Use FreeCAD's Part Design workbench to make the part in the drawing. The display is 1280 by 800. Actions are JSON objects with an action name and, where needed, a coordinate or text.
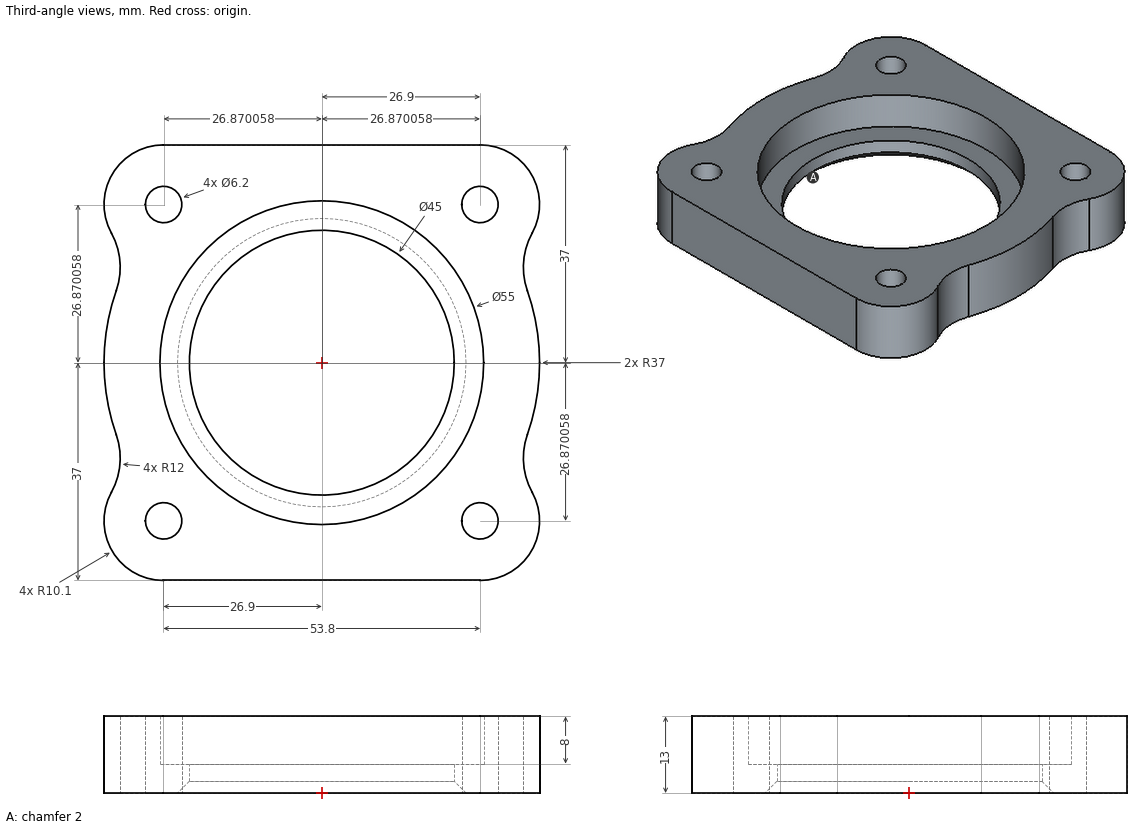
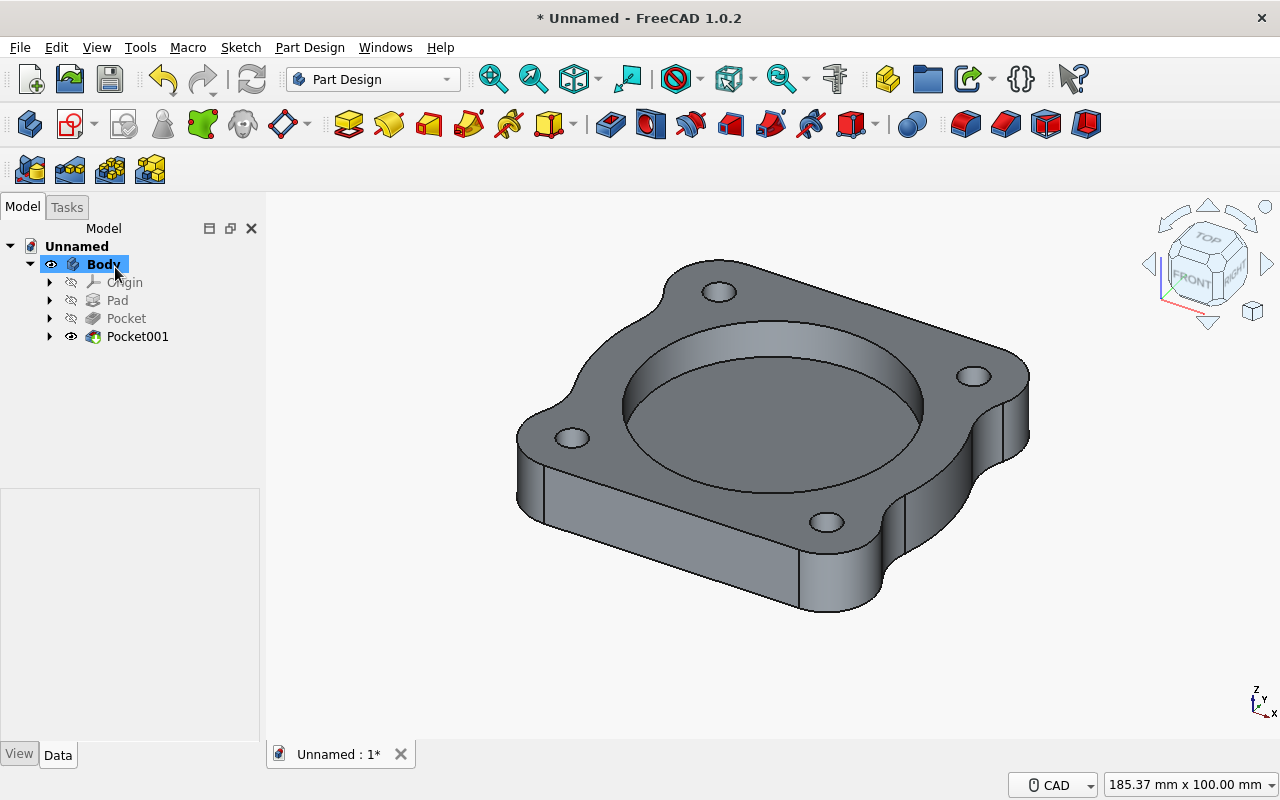
{"action": "left_click", "coordinate": [773, 442]}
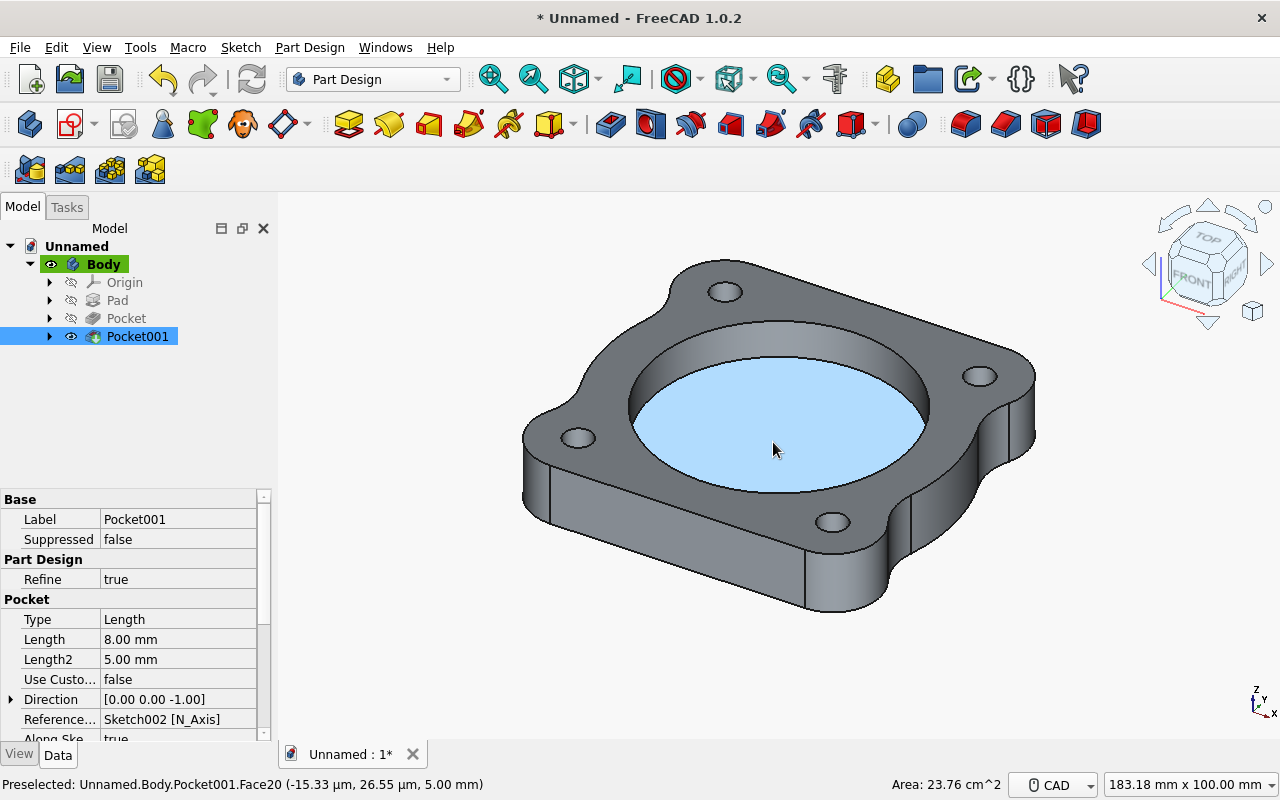
{"action": "left_click", "coordinate": [70, 124]}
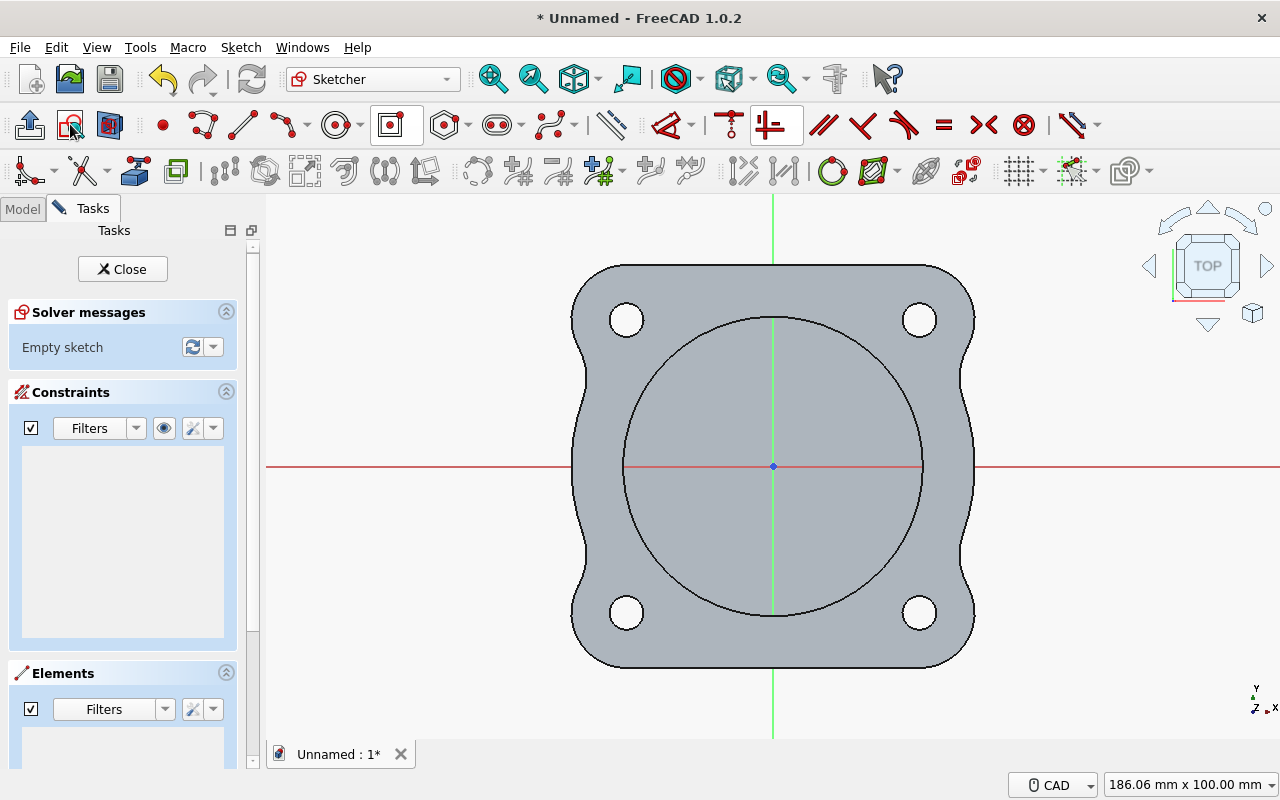
{"action": "left_click", "coordinate": [110, 126]}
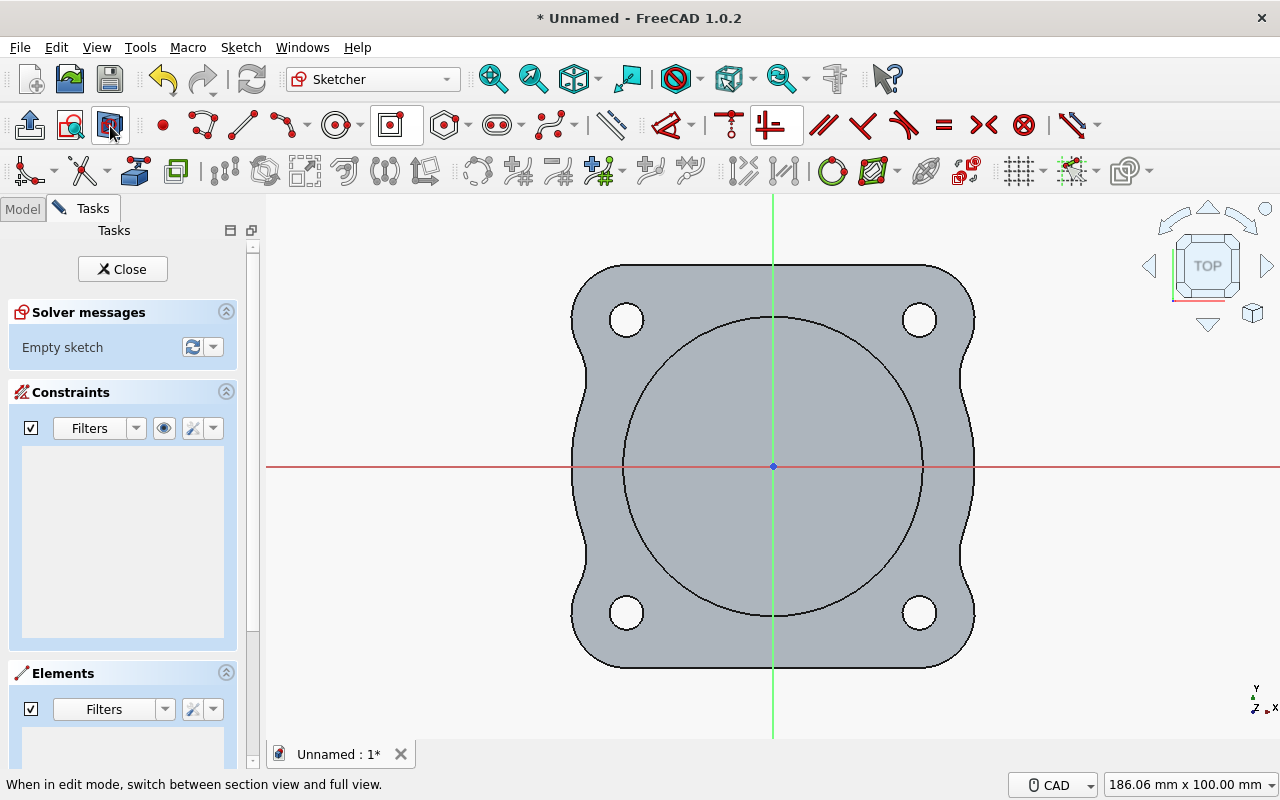
{"action": "scroll", "coordinate": [912, 467], "scroll_direction": "up", "scroll_amount": 2}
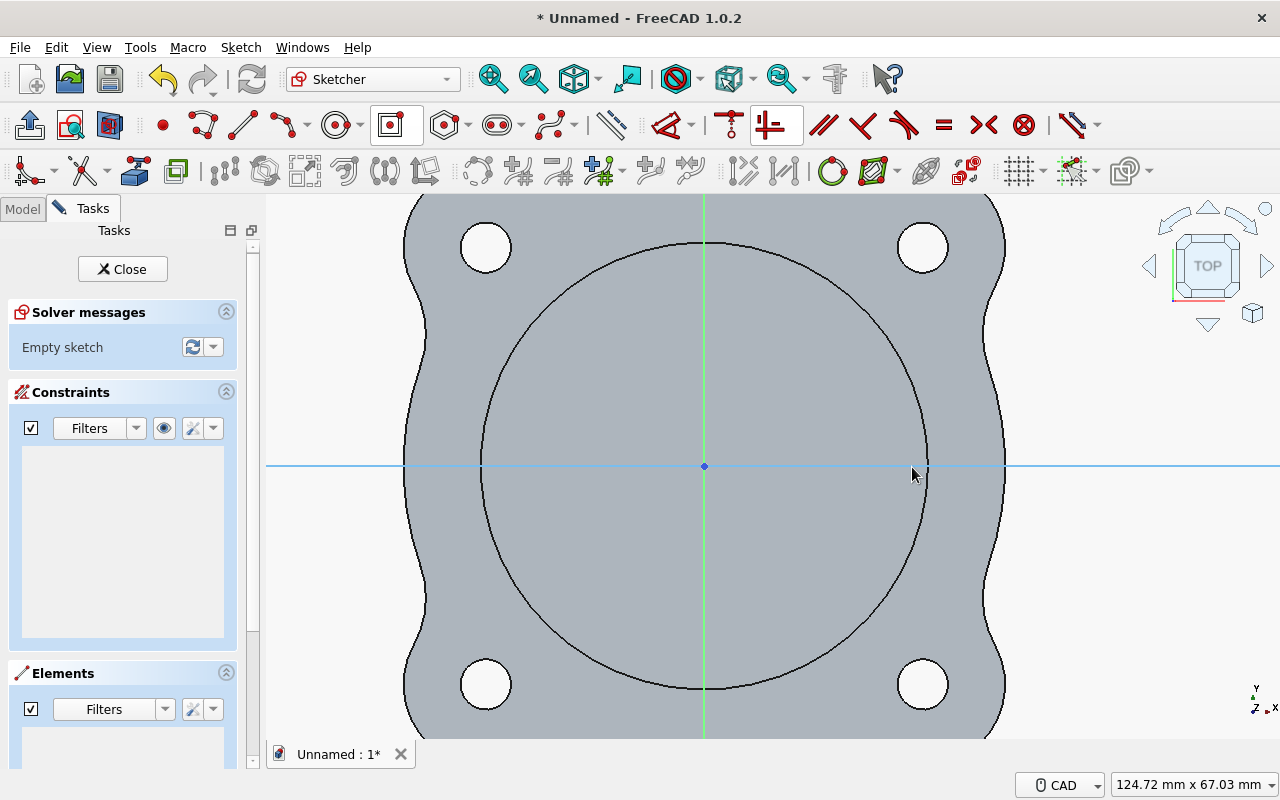
{"action": "key", "text": "g c"}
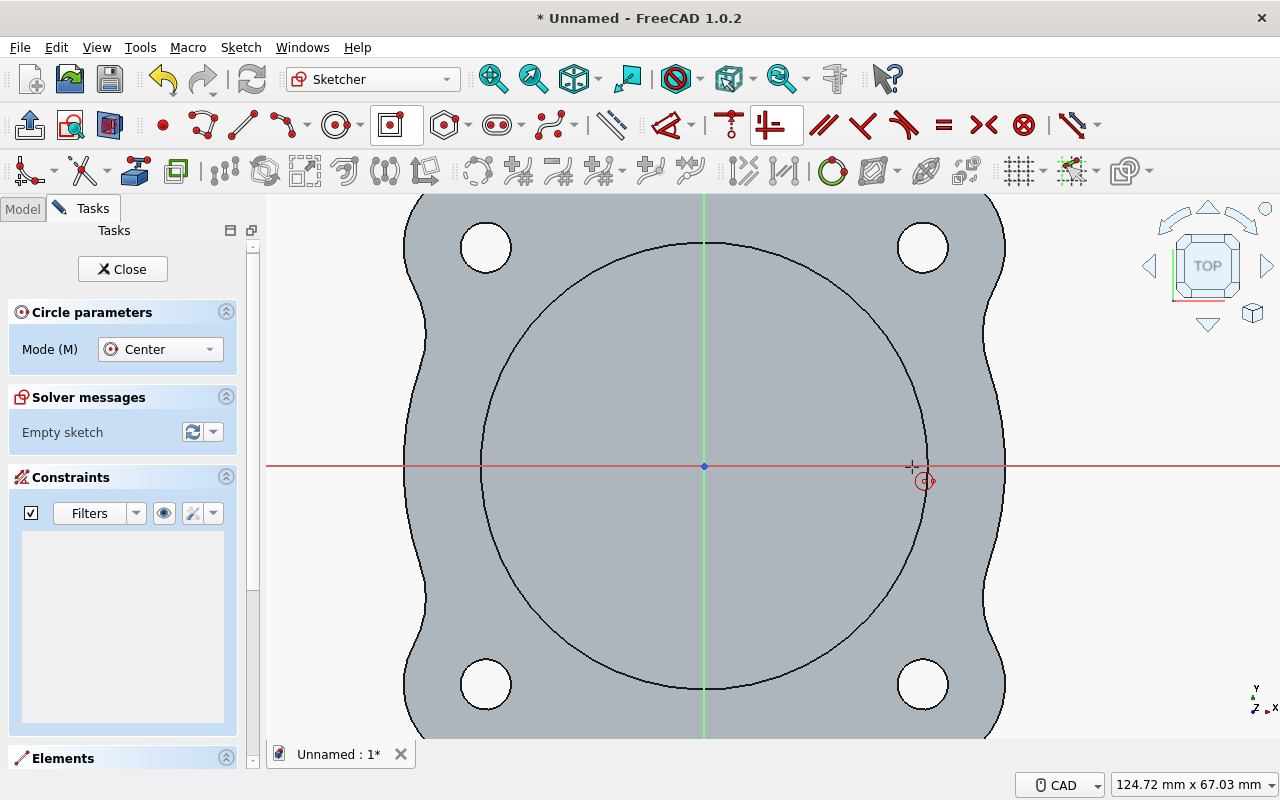
{"action": "left_click", "coordinate": [704, 466]}
{"action": "left_click", "coordinate": [834, 337]}
{"action": "key", "text": "Escape"}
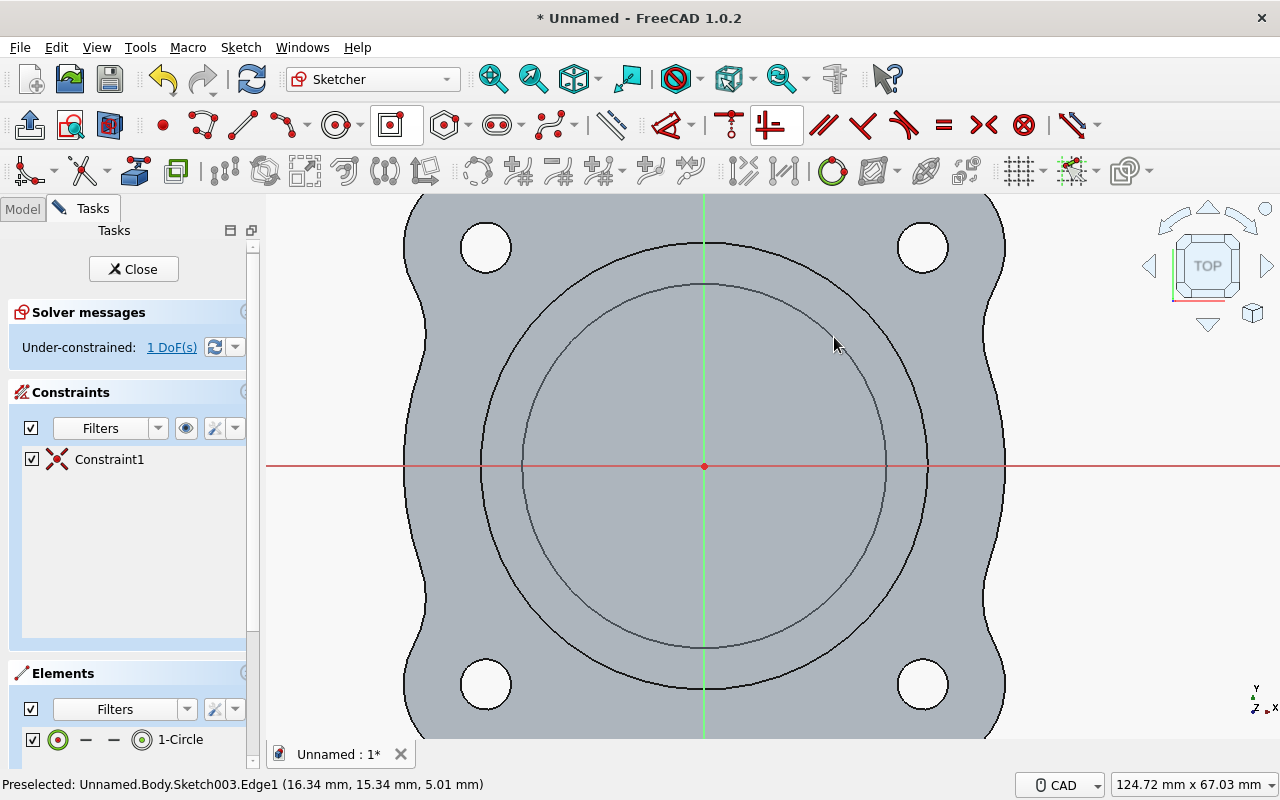
{"action": "key", "text": "d"}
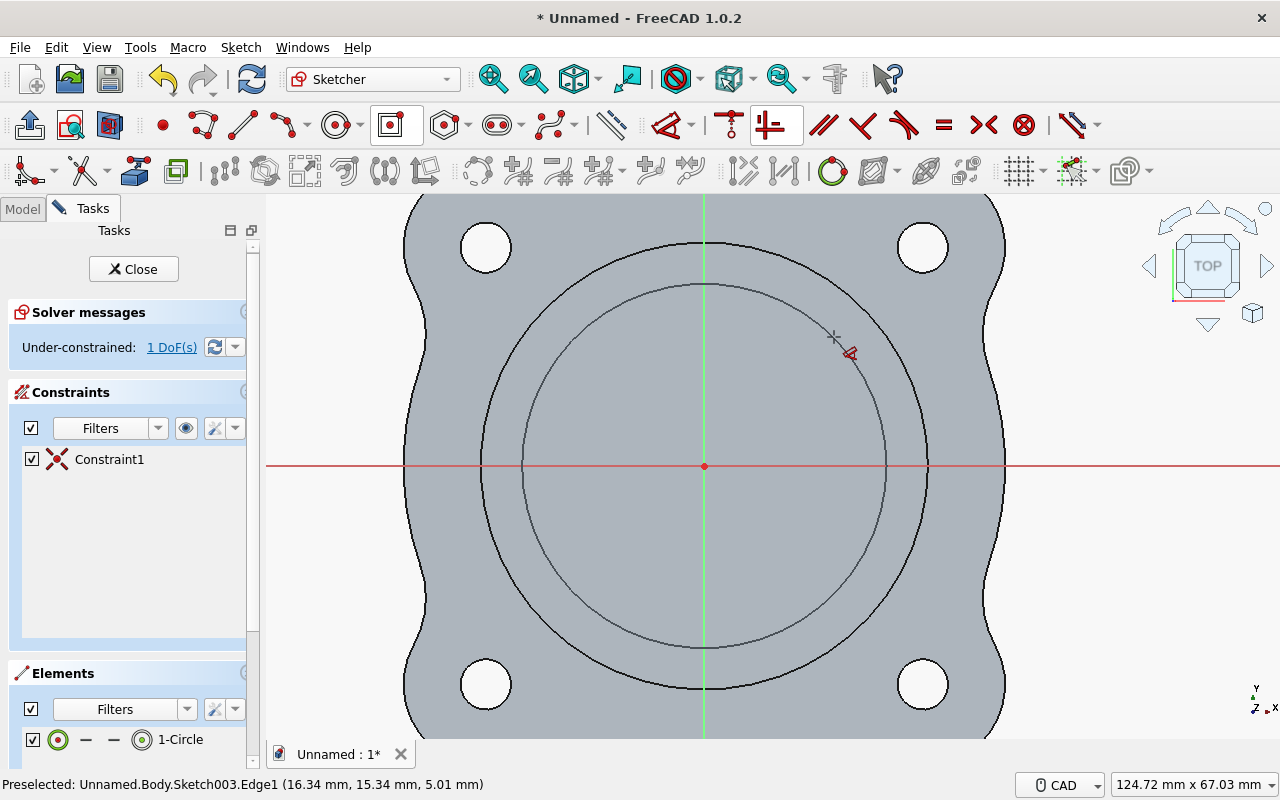
{"action": "left_click", "coordinate": [833, 337]}
{"action": "left_click", "coordinate": [856, 314]}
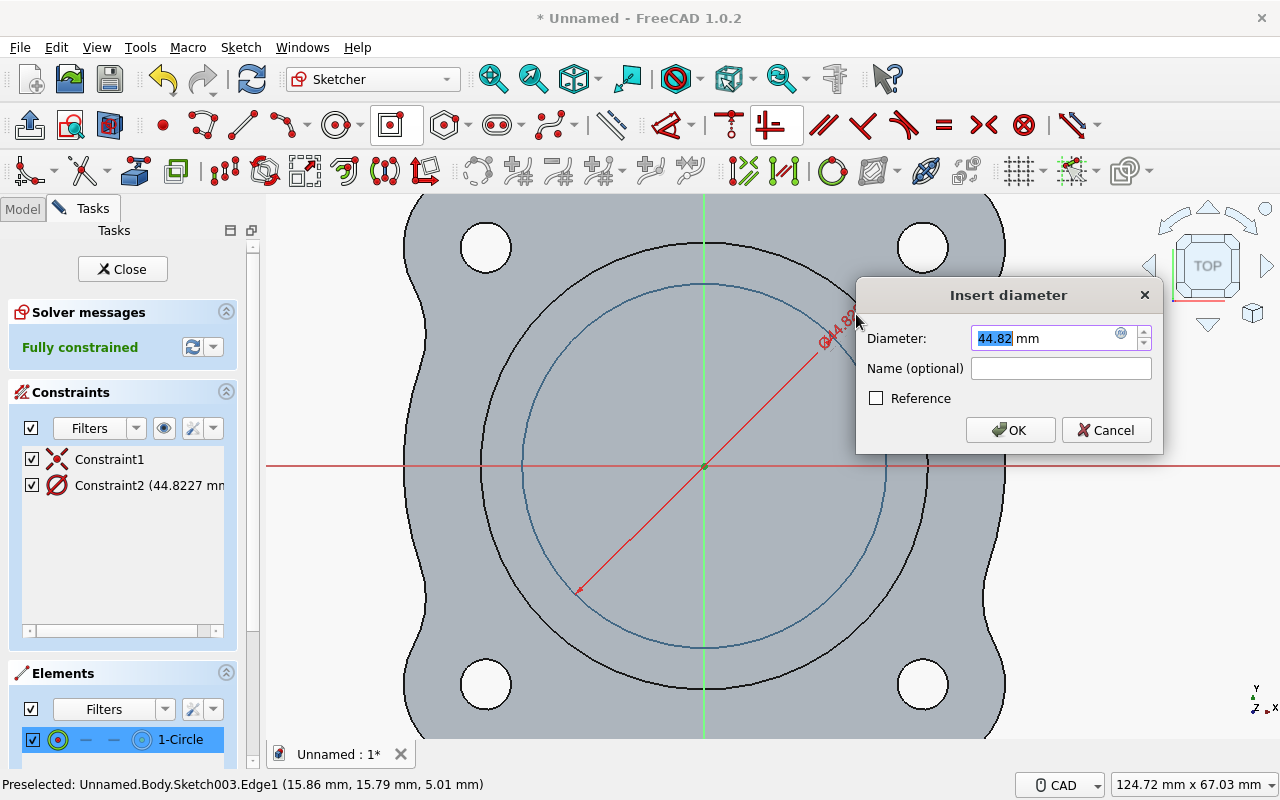
{"action": "type", "text": "45"}
{"action": "key", "text": "Return"}
{"action": "key", "text": "Escape"}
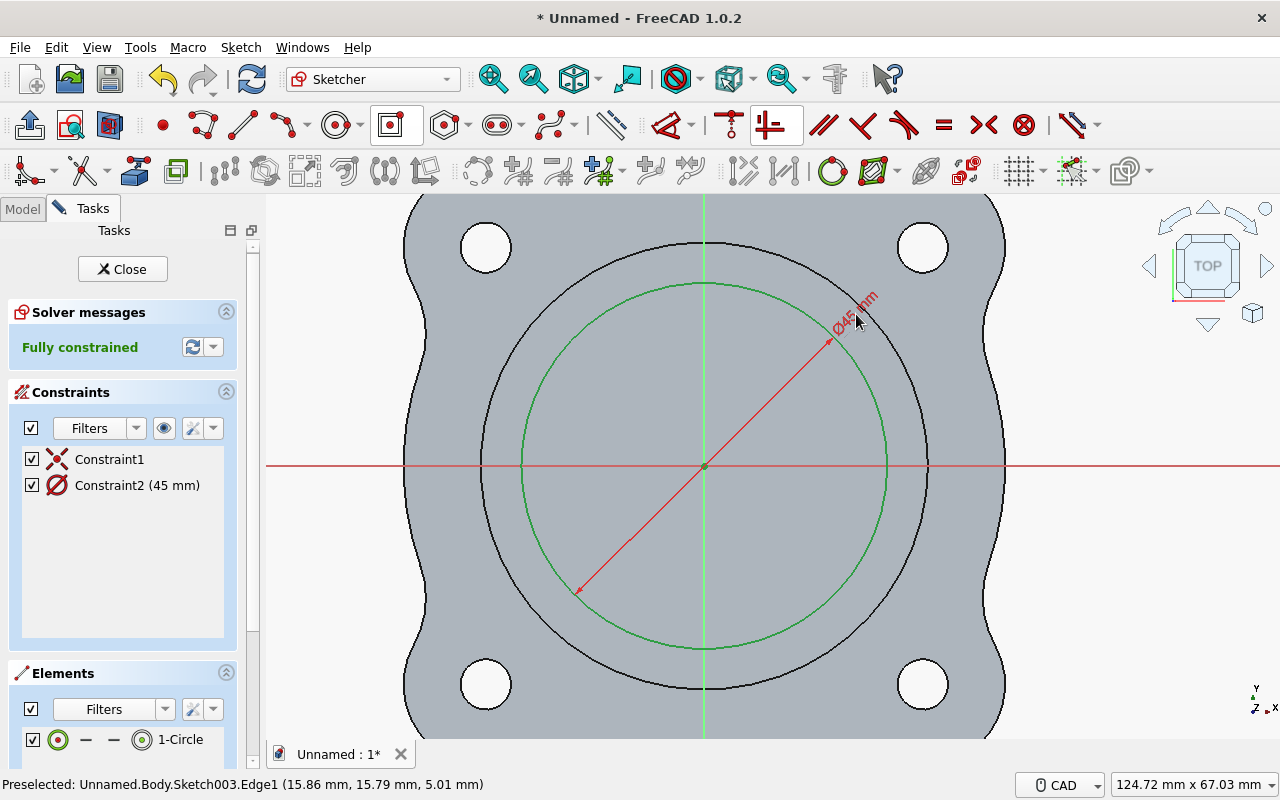
{"action": "left_click", "coordinate": [123, 269]}